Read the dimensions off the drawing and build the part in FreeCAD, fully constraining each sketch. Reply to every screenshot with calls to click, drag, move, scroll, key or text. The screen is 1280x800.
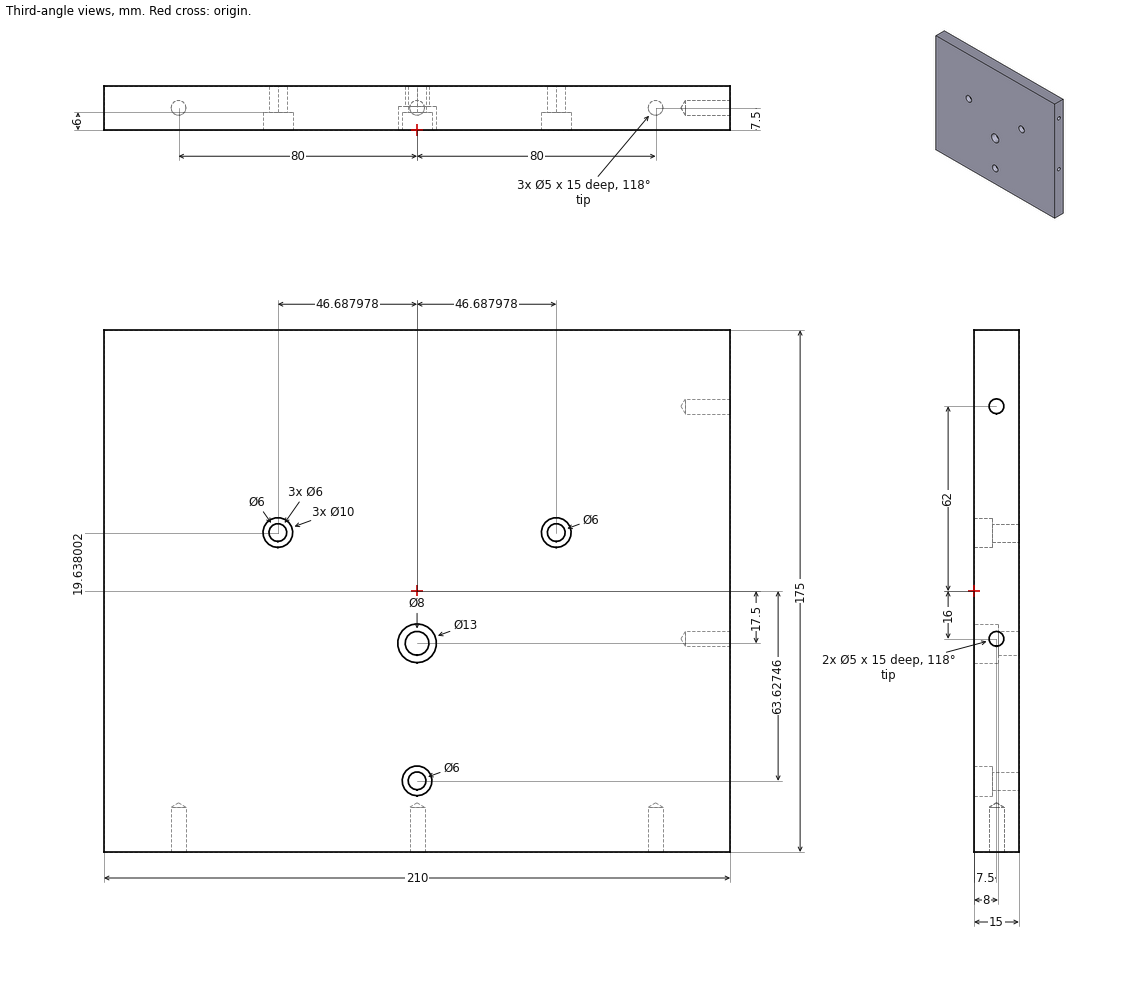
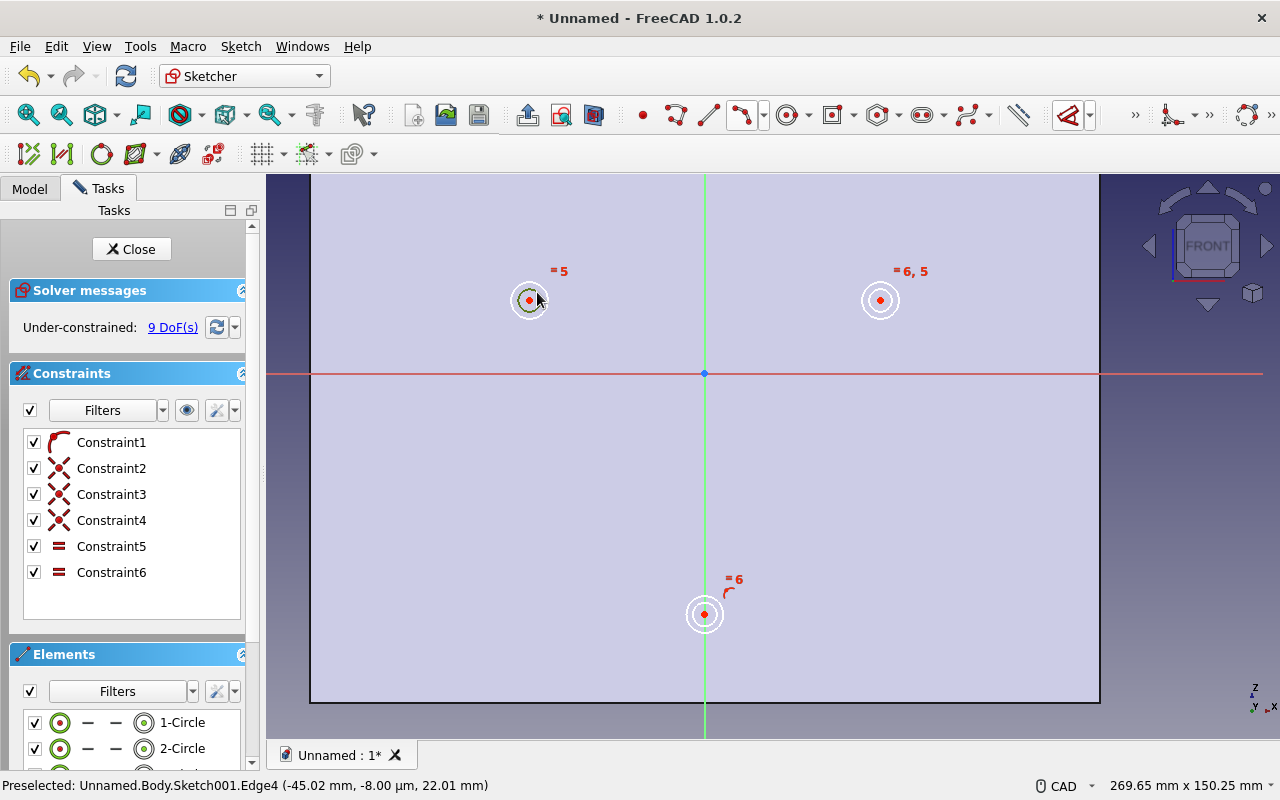
scroll(888, 293, up, 4)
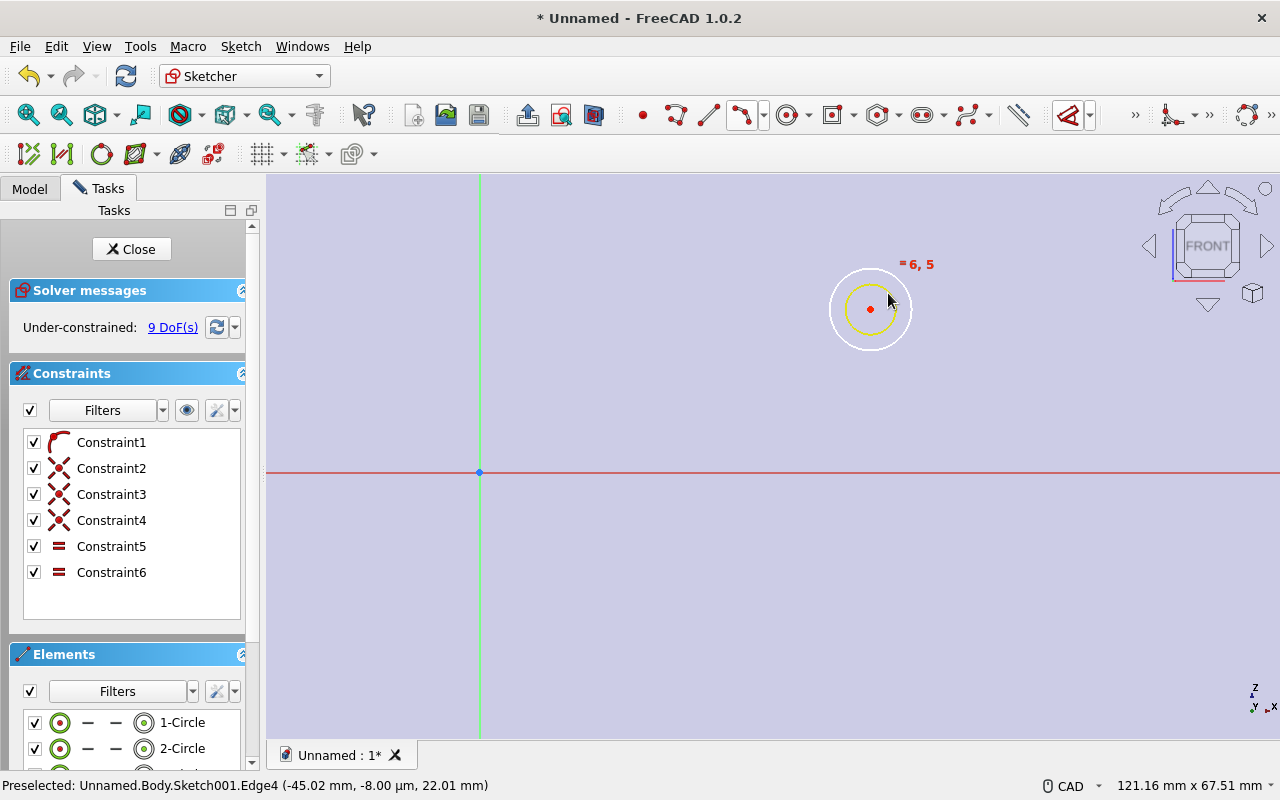
click(888, 292)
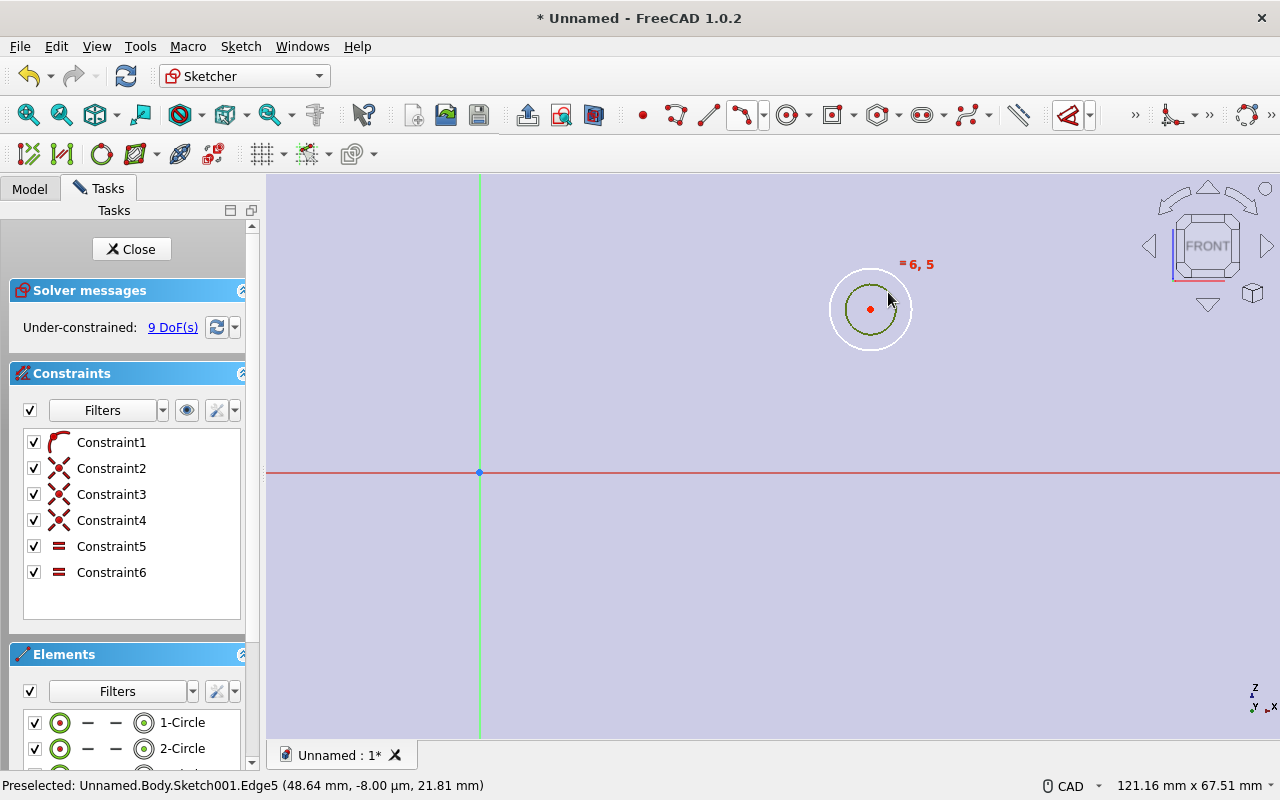
scroll(888, 293, down, 4)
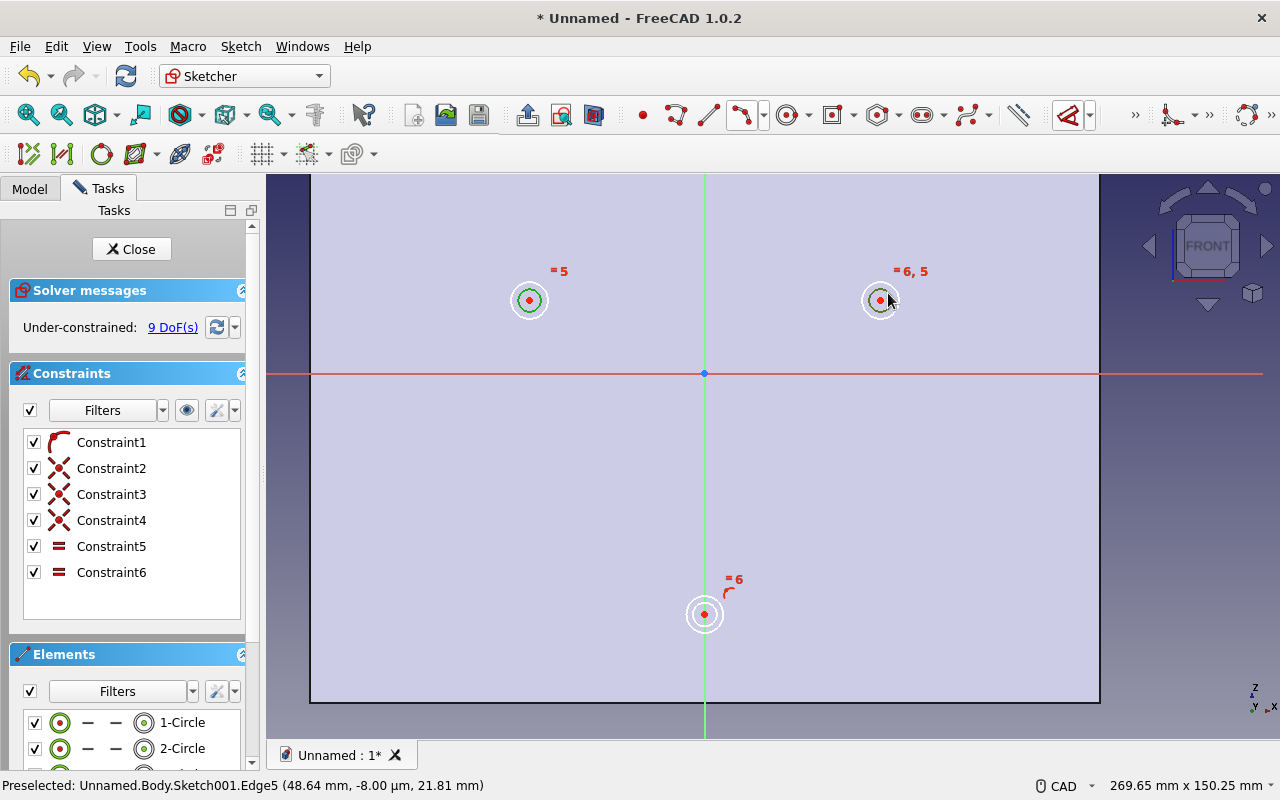
scroll(713, 606, up, 4)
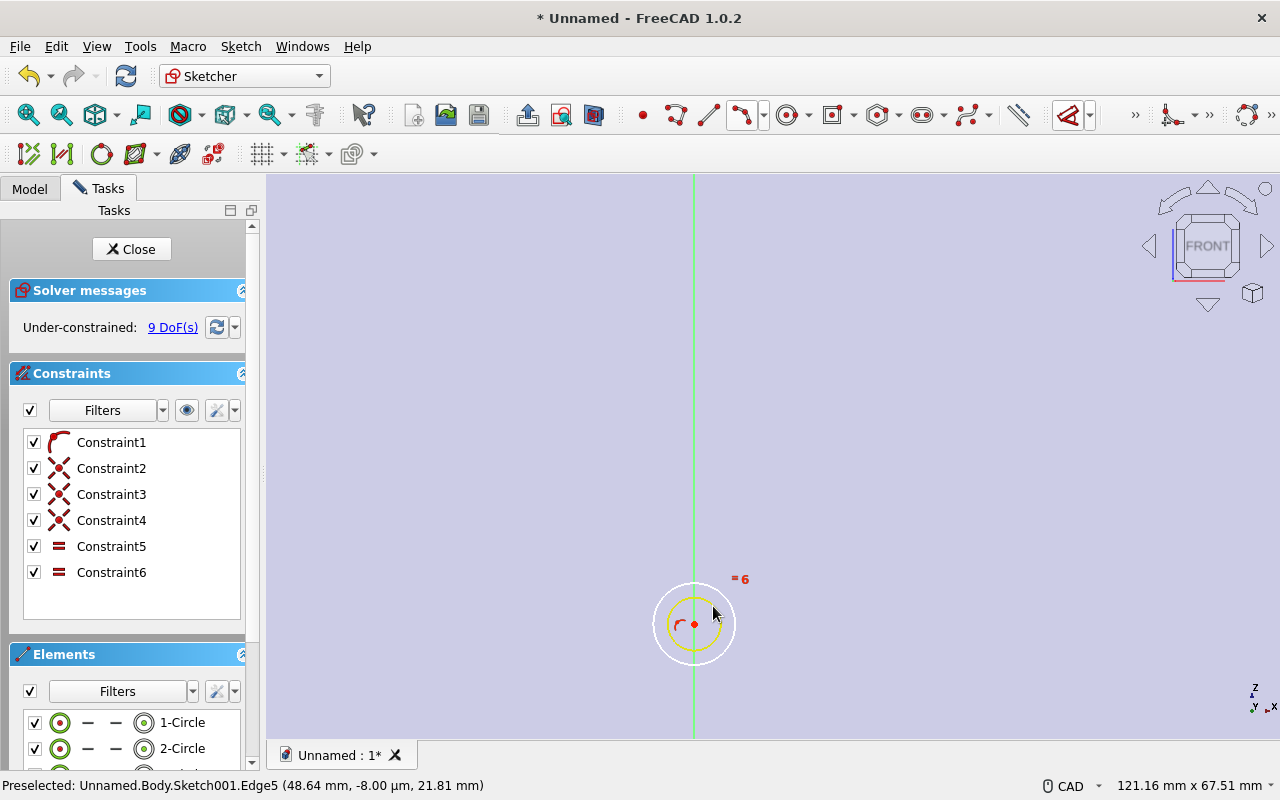
click(713, 605)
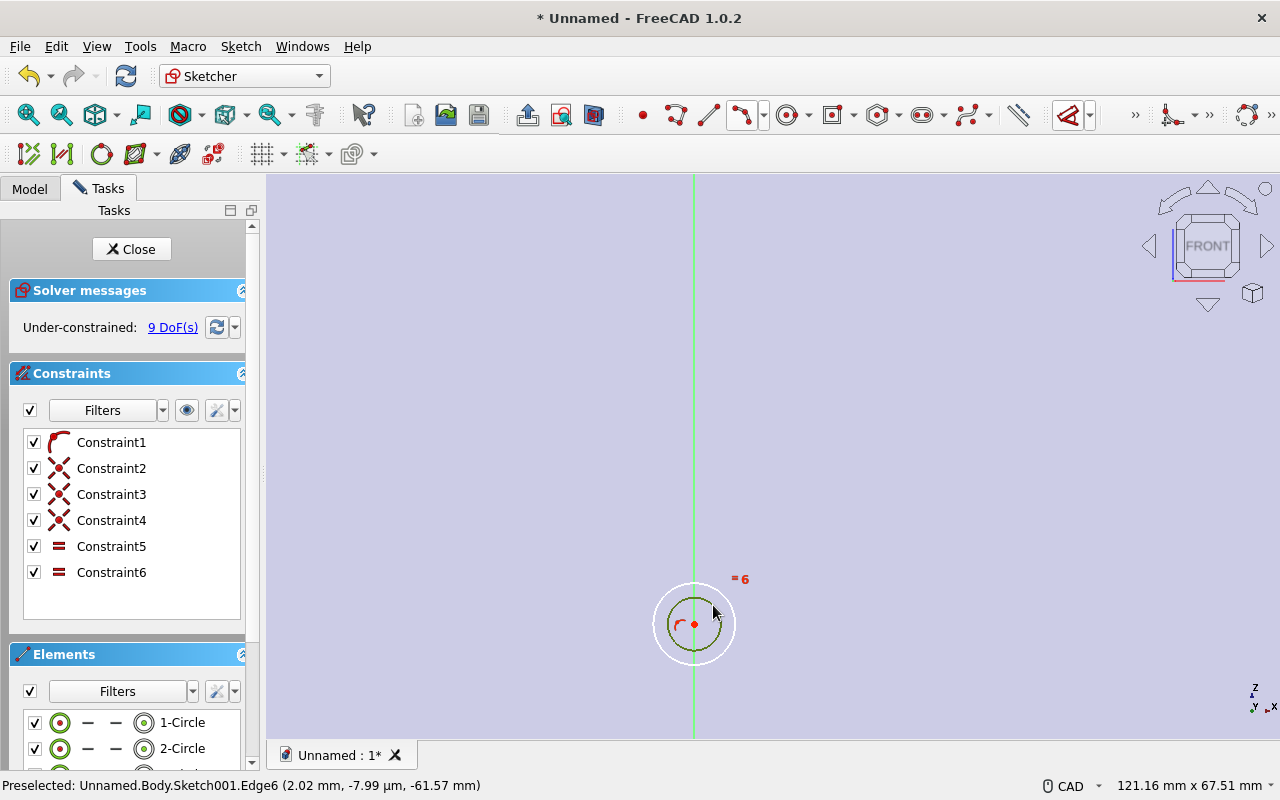
key(e)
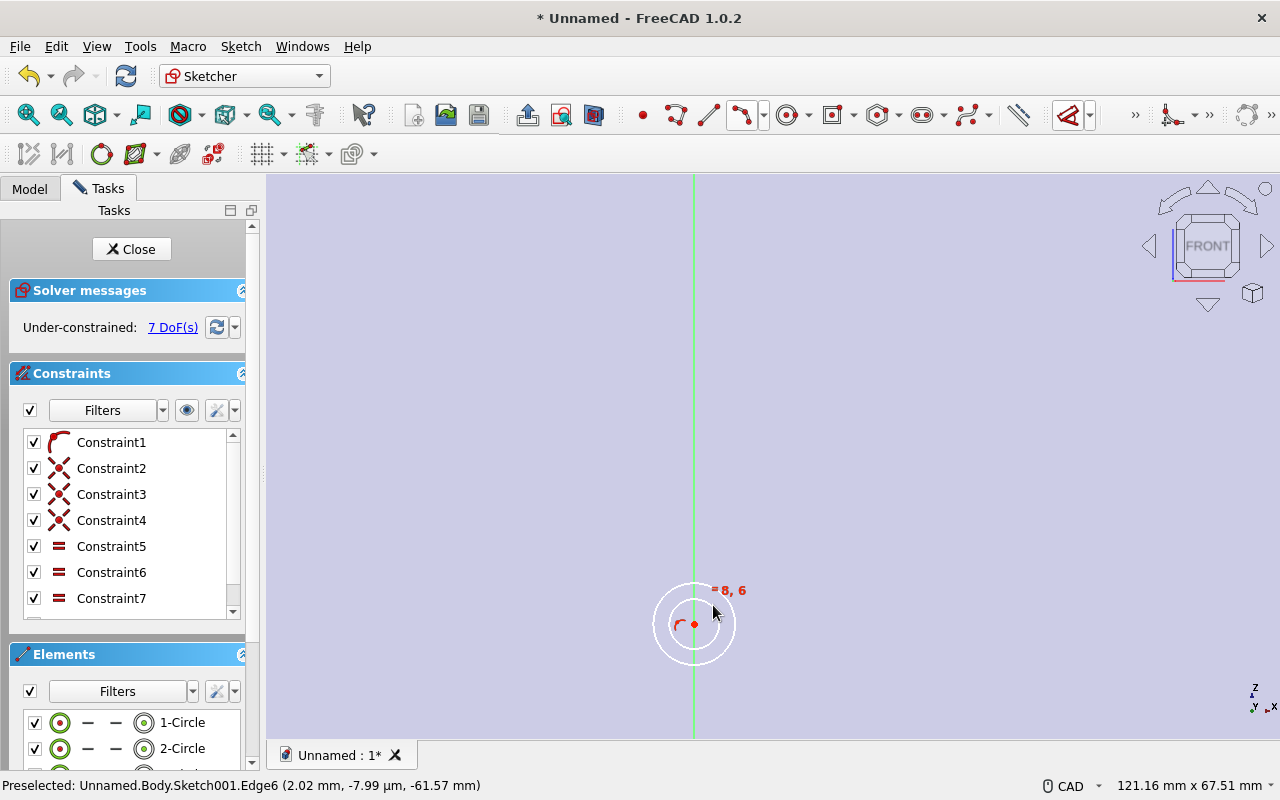
scroll(713, 607, down, 4)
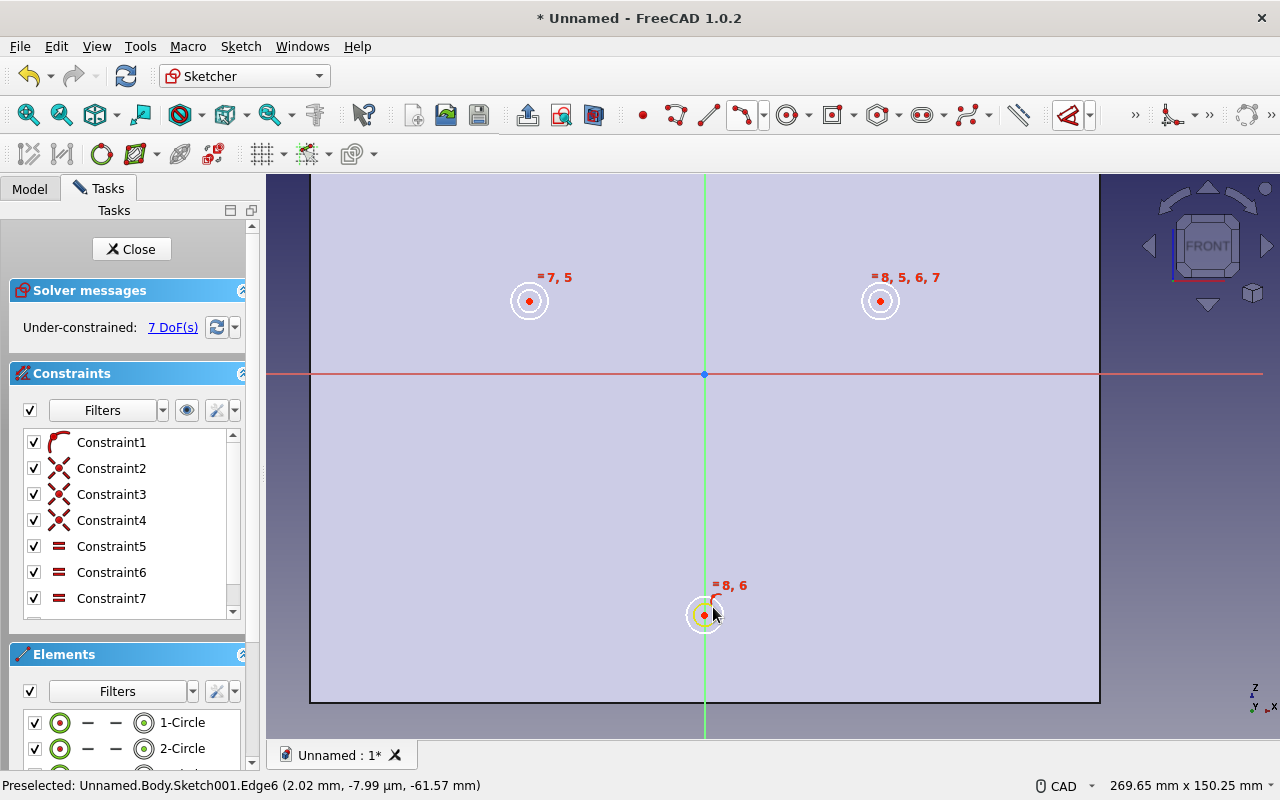
click(530, 301)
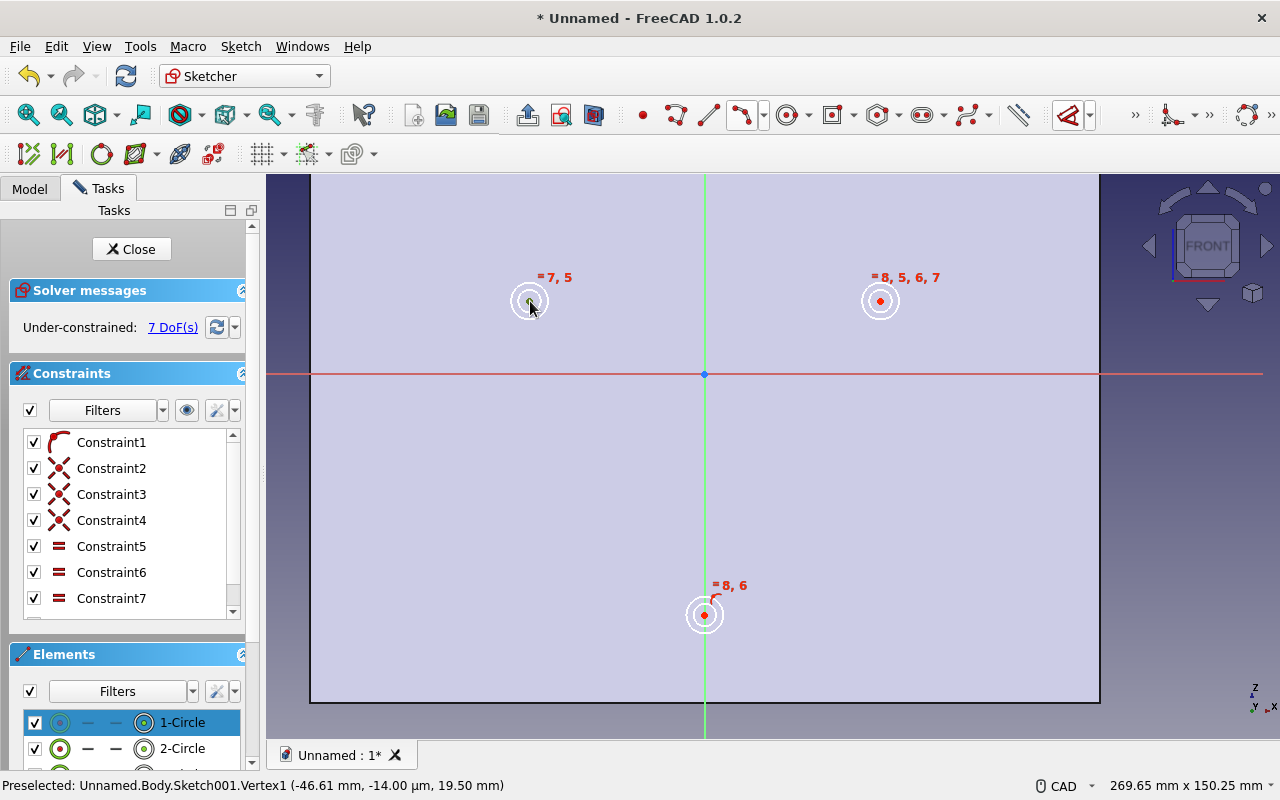
click(881, 301)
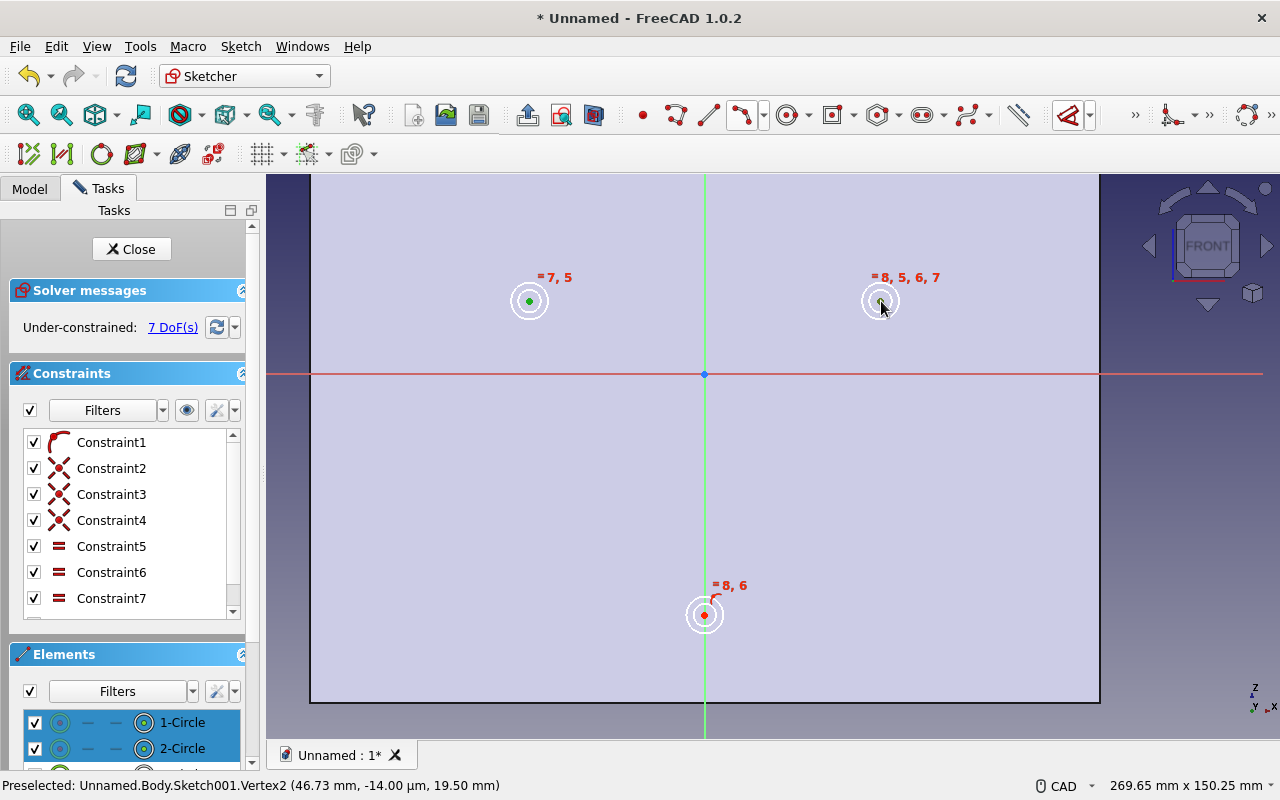
key(h)